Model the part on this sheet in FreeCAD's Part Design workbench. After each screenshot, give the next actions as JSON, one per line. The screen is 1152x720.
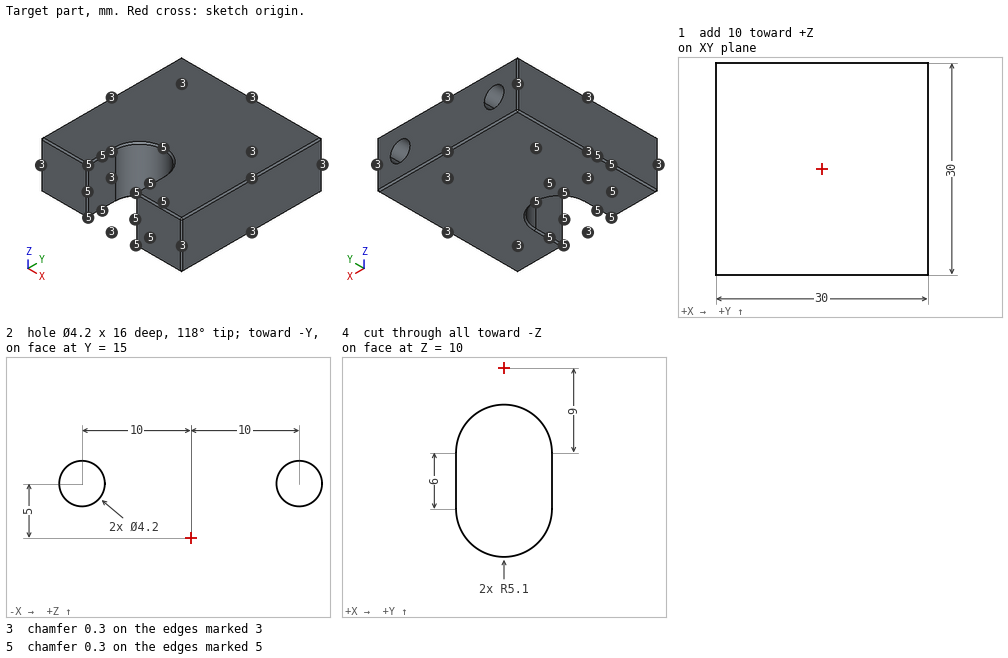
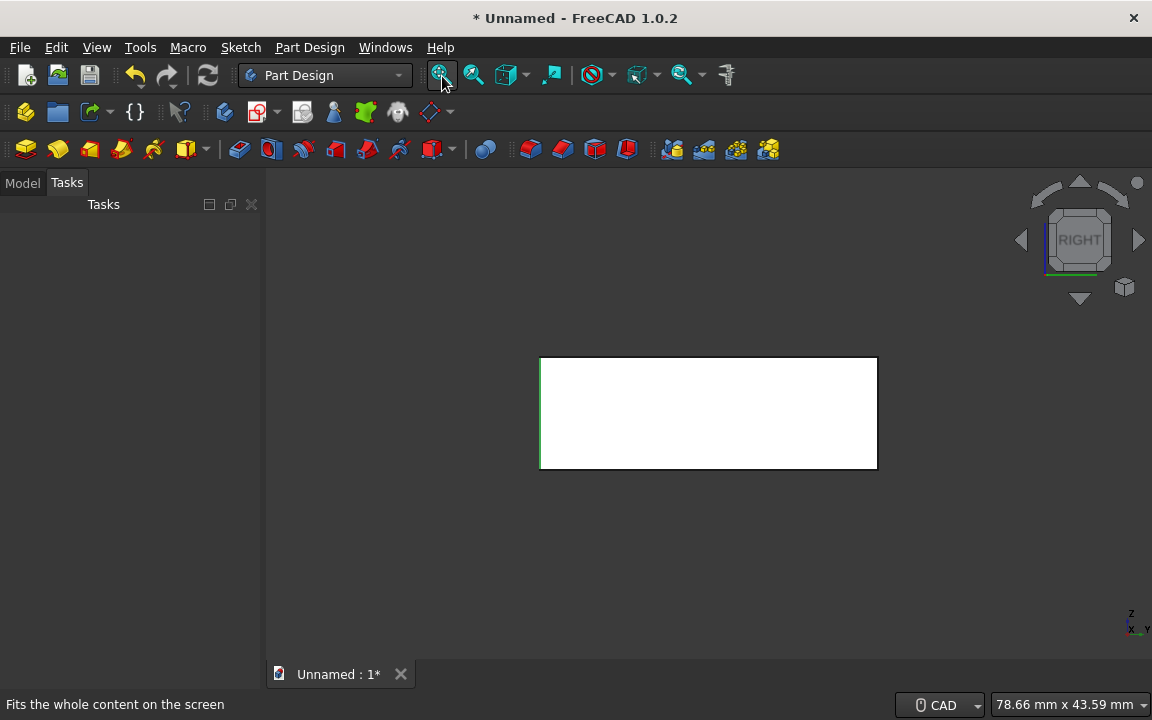
{"action": "left_click", "coordinate": [878, 412], "text": "ctrl"}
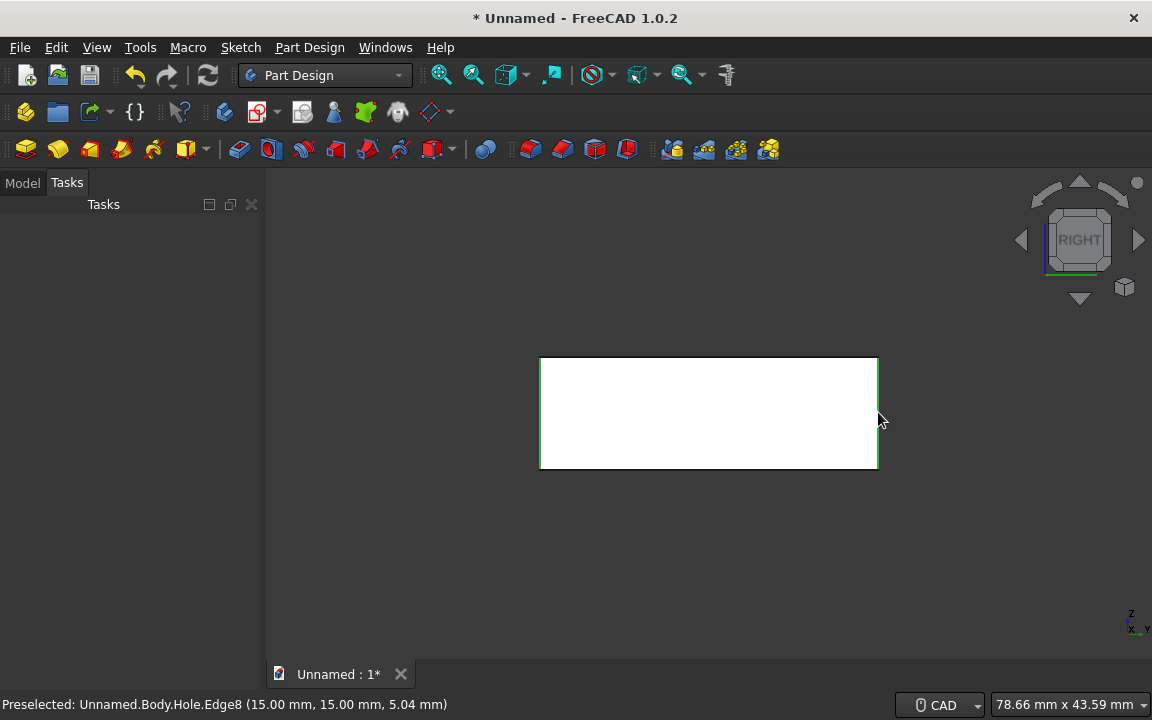
{"action": "key", "text": "5"}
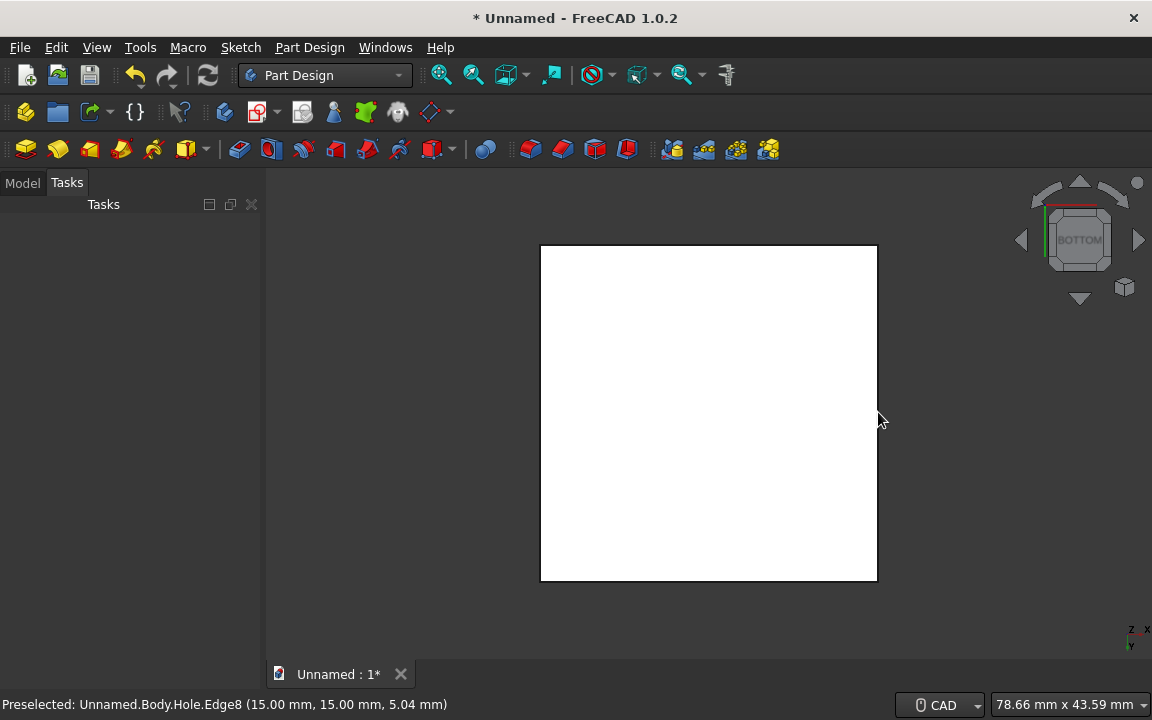
{"action": "left_click", "coordinate": [709, 412], "text": "ctrl"}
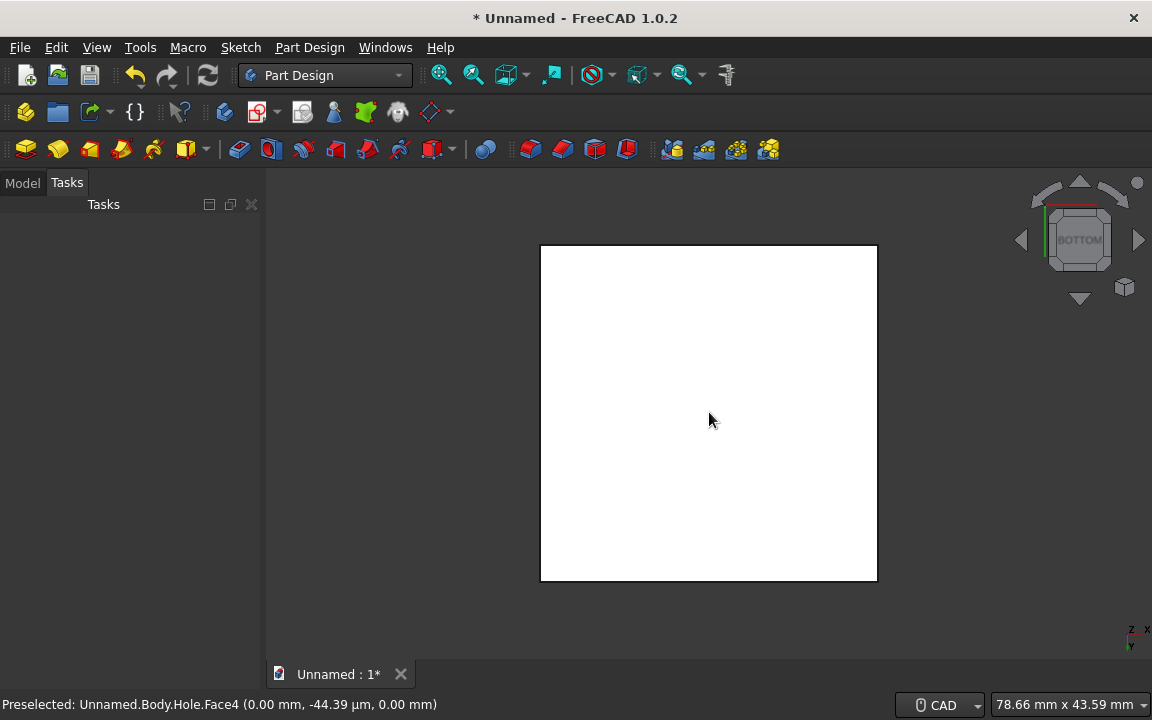
{"action": "left_click", "coordinate": [564, 150]}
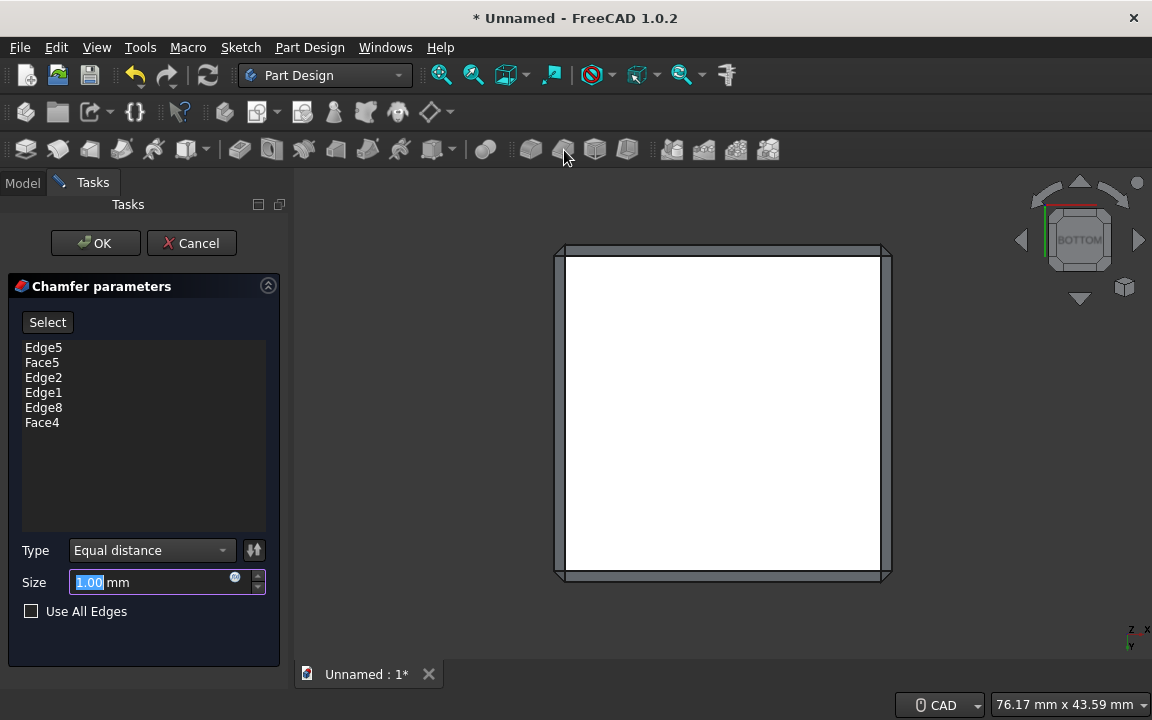
{"action": "type", "text": "0.3"}
{"action": "key", "text": "Tab"}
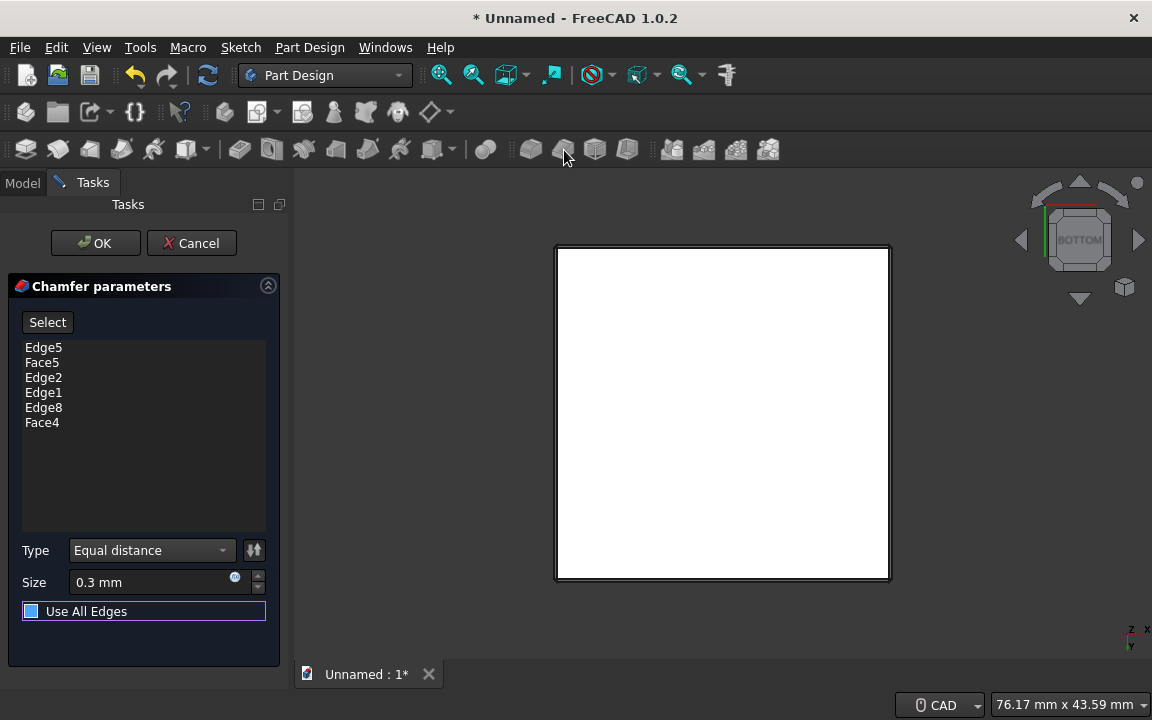
{"action": "left_click", "coordinate": [96, 243]}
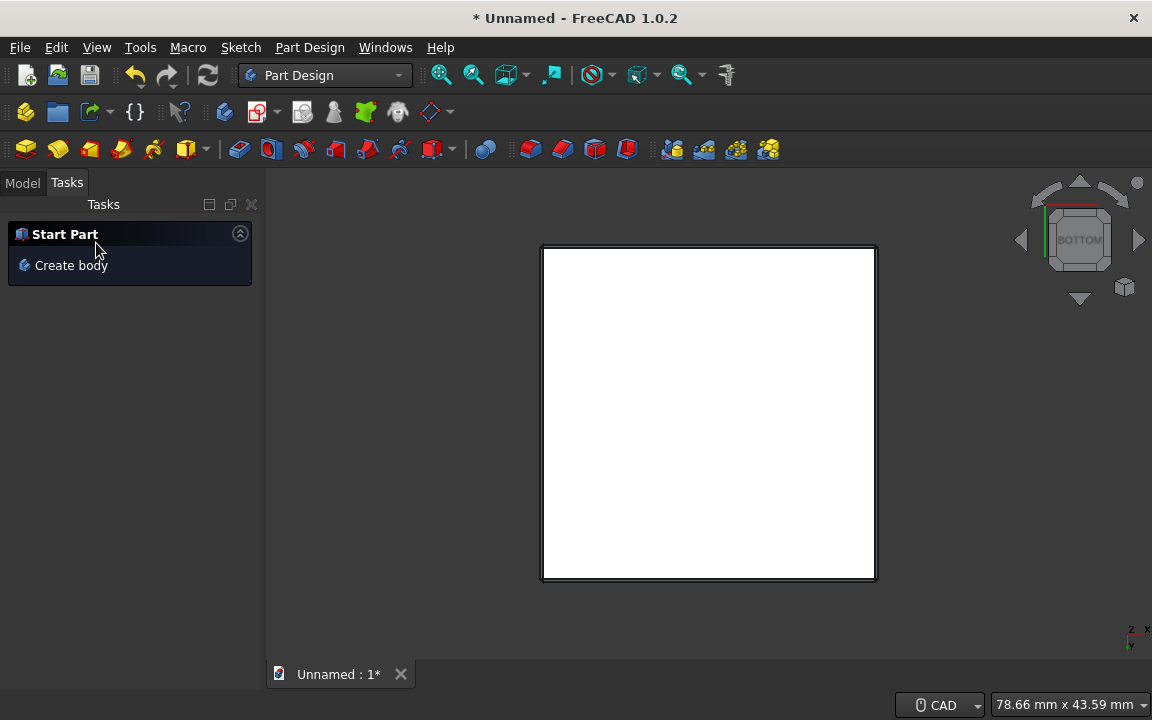
{"action": "key", "text": "0"}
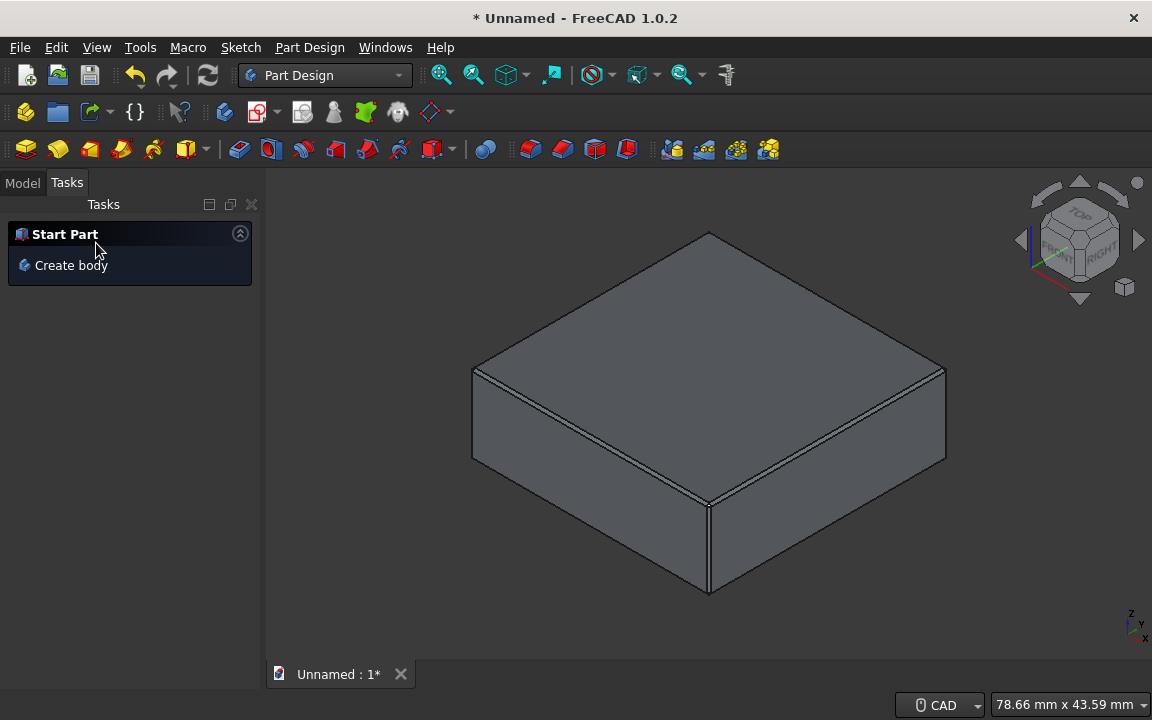
{"action": "left_click", "coordinate": [709, 367]}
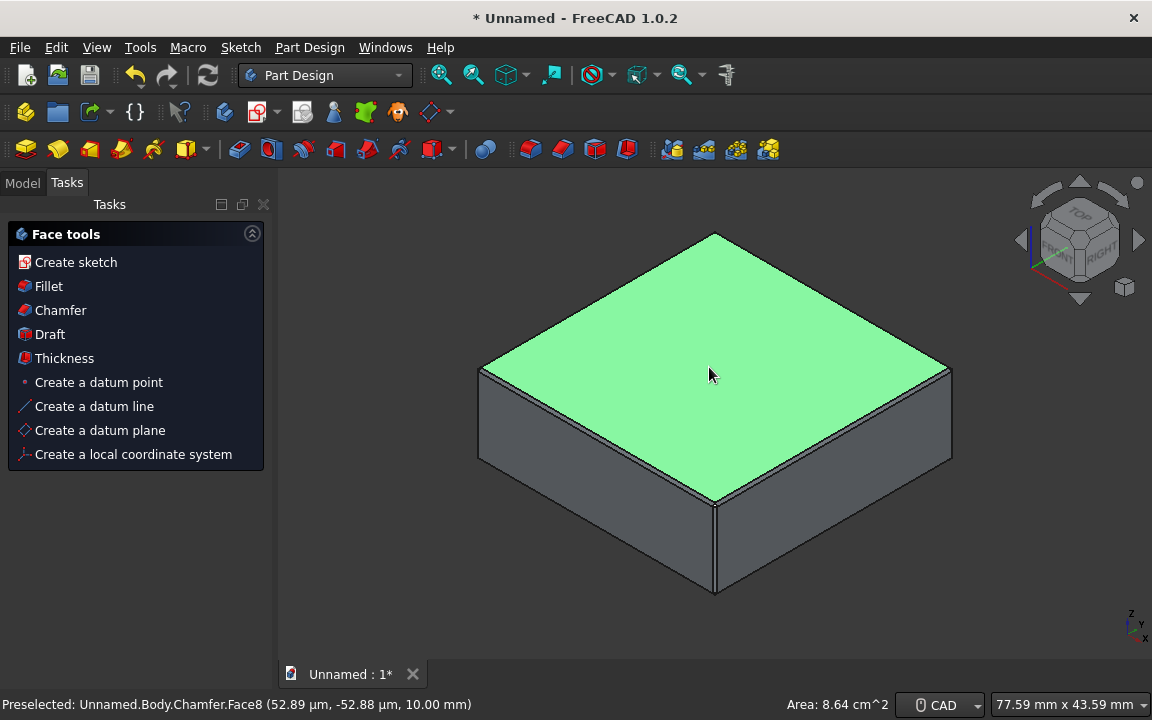
{"action": "left_click", "coordinate": [258, 112]}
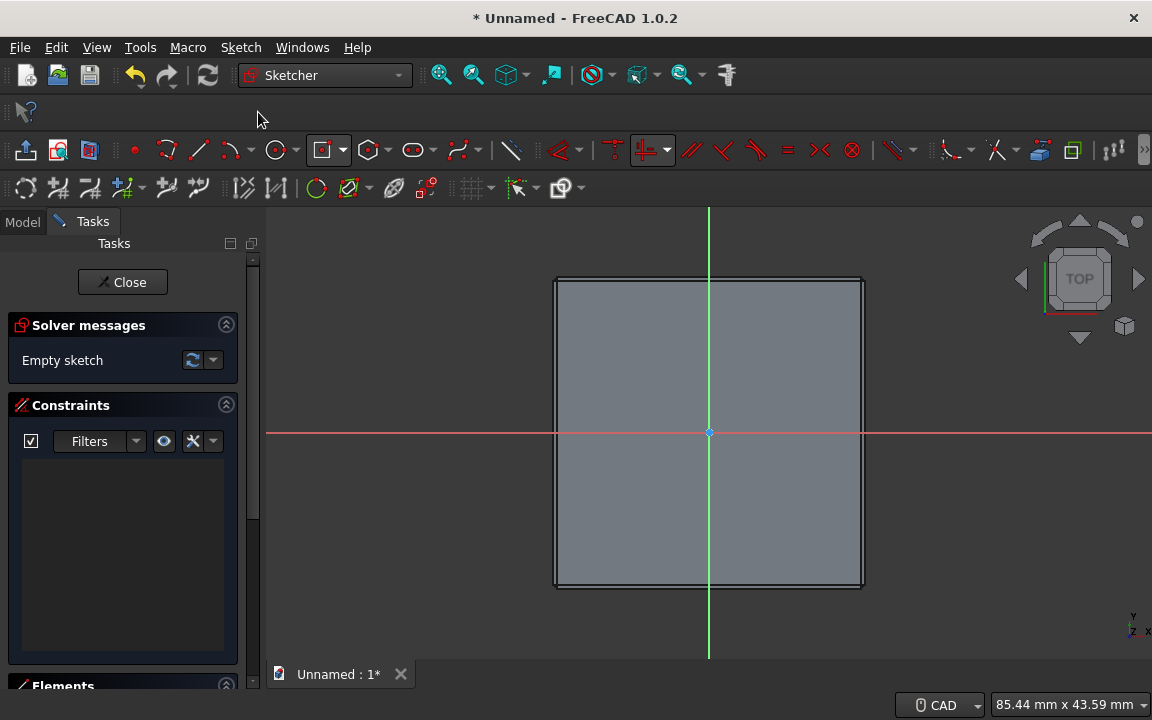
{"action": "scroll", "coordinate": [331, 235], "scroll_direction": "down", "scroll_amount": 1}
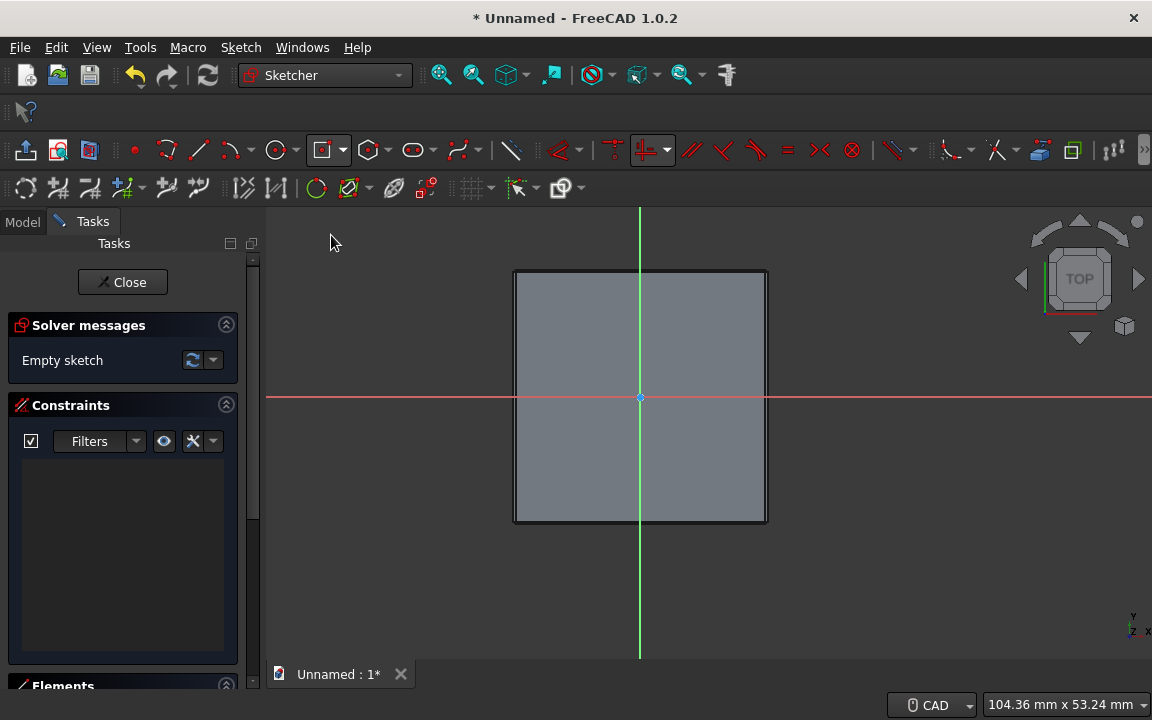
{"action": "scroll", "coordinate": [640, 583], "scroll_direction": "up", "scroll_amount": 2}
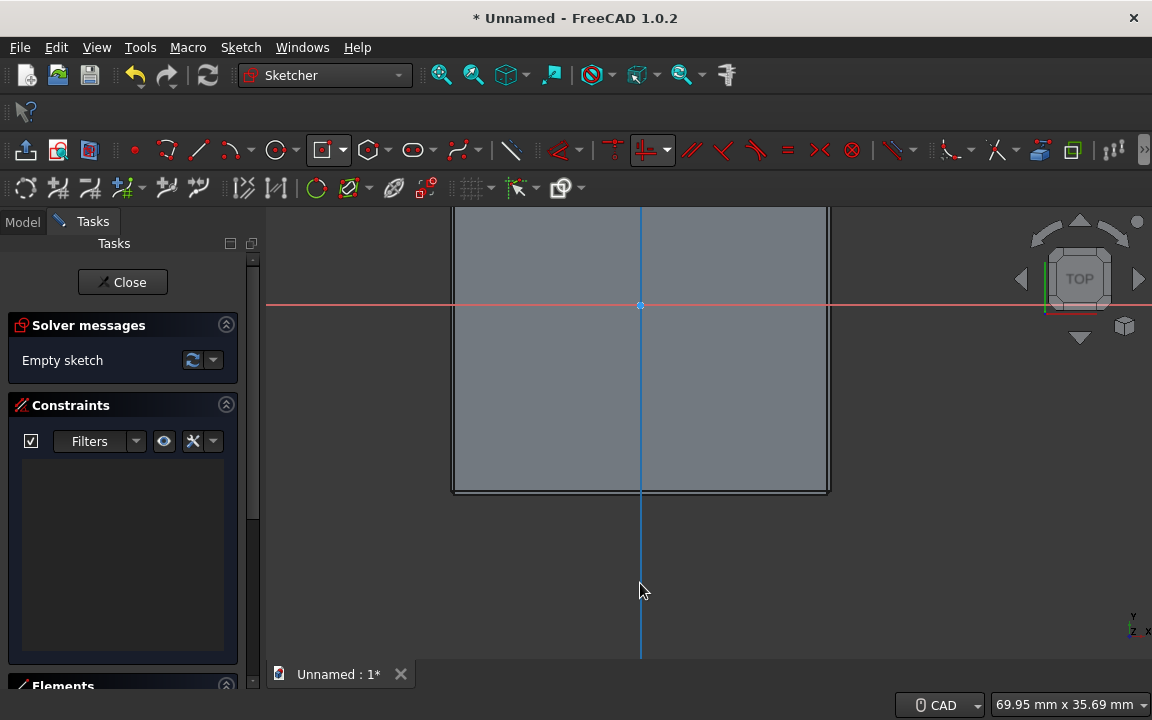
{"action": "left_click", "coordinate": [414, 150]}